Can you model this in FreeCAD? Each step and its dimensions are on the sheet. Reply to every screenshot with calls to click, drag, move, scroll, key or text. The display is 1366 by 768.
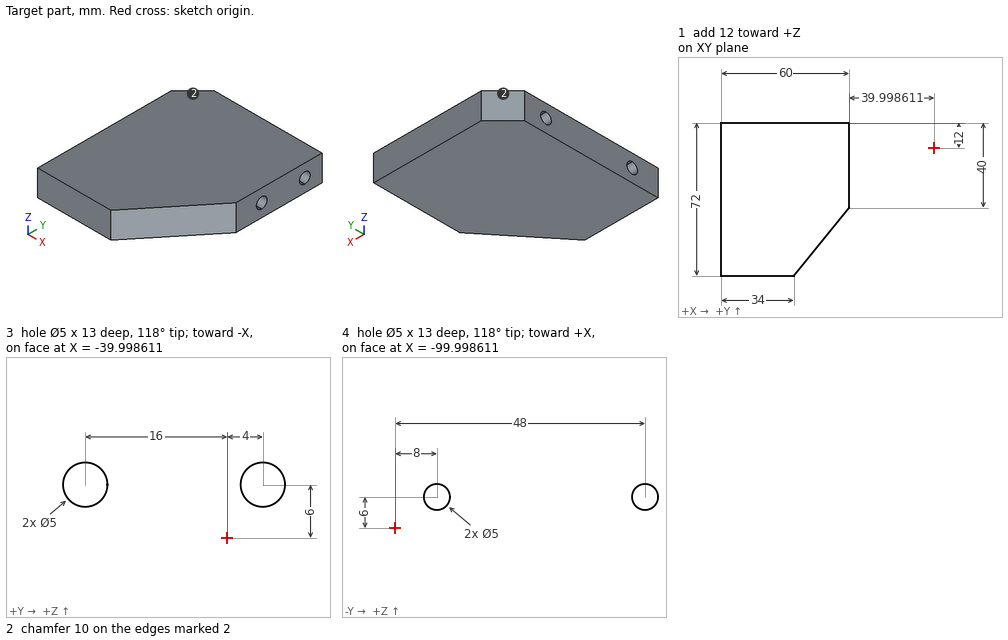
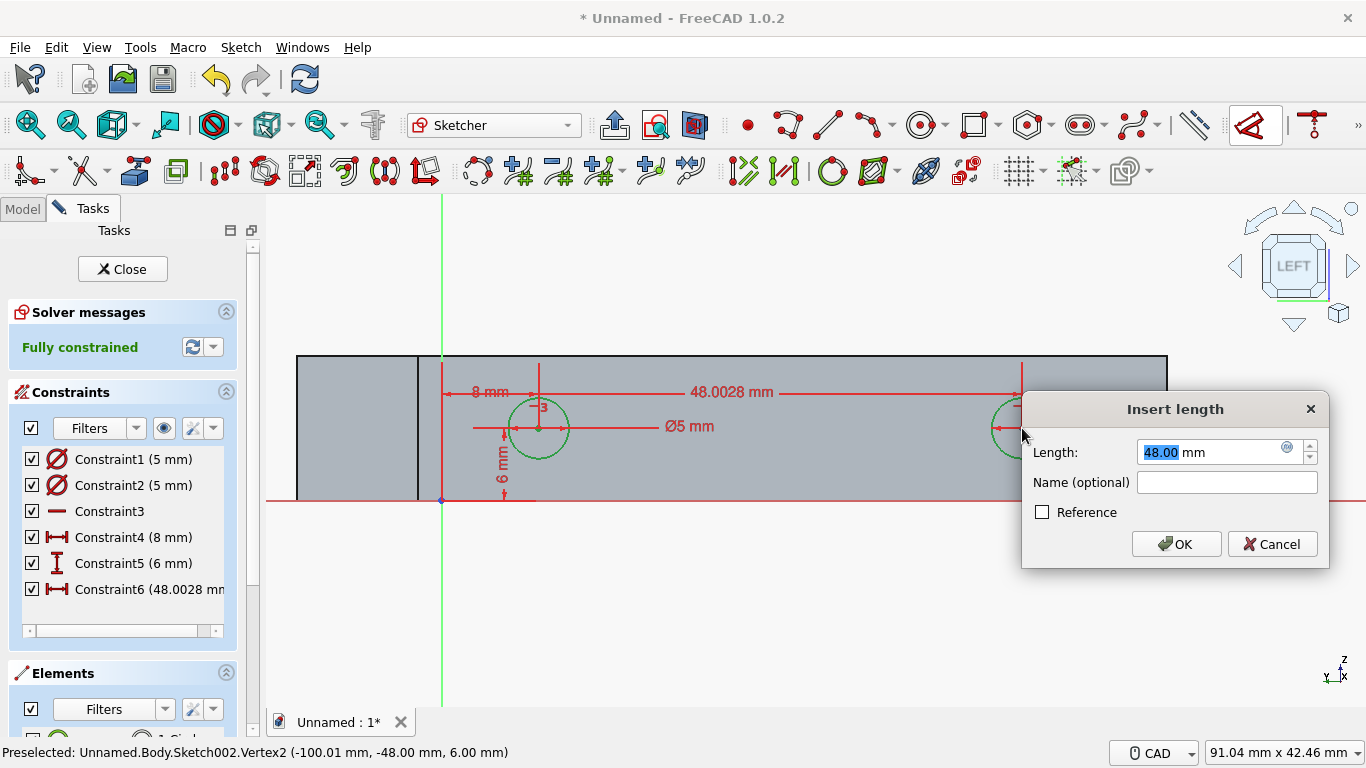
text(48)
key(Return)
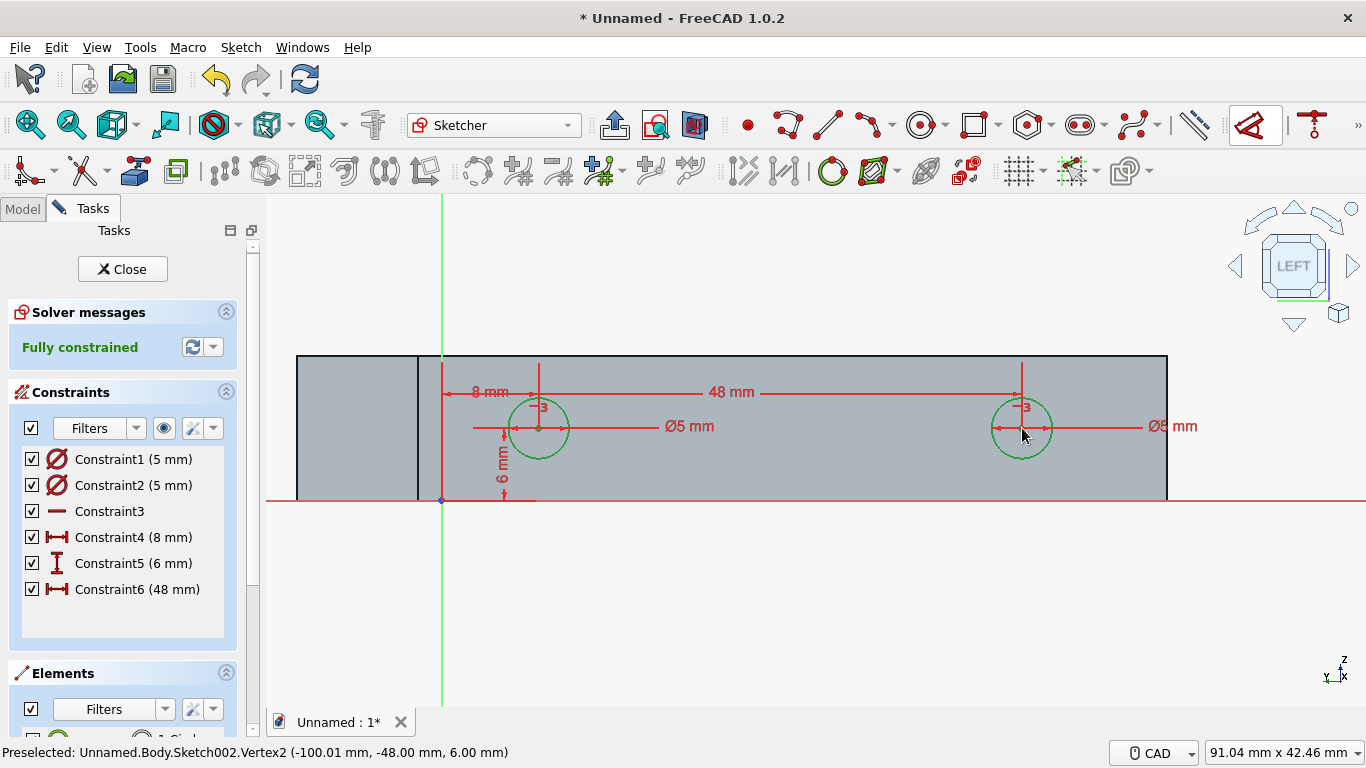
click(123, 269)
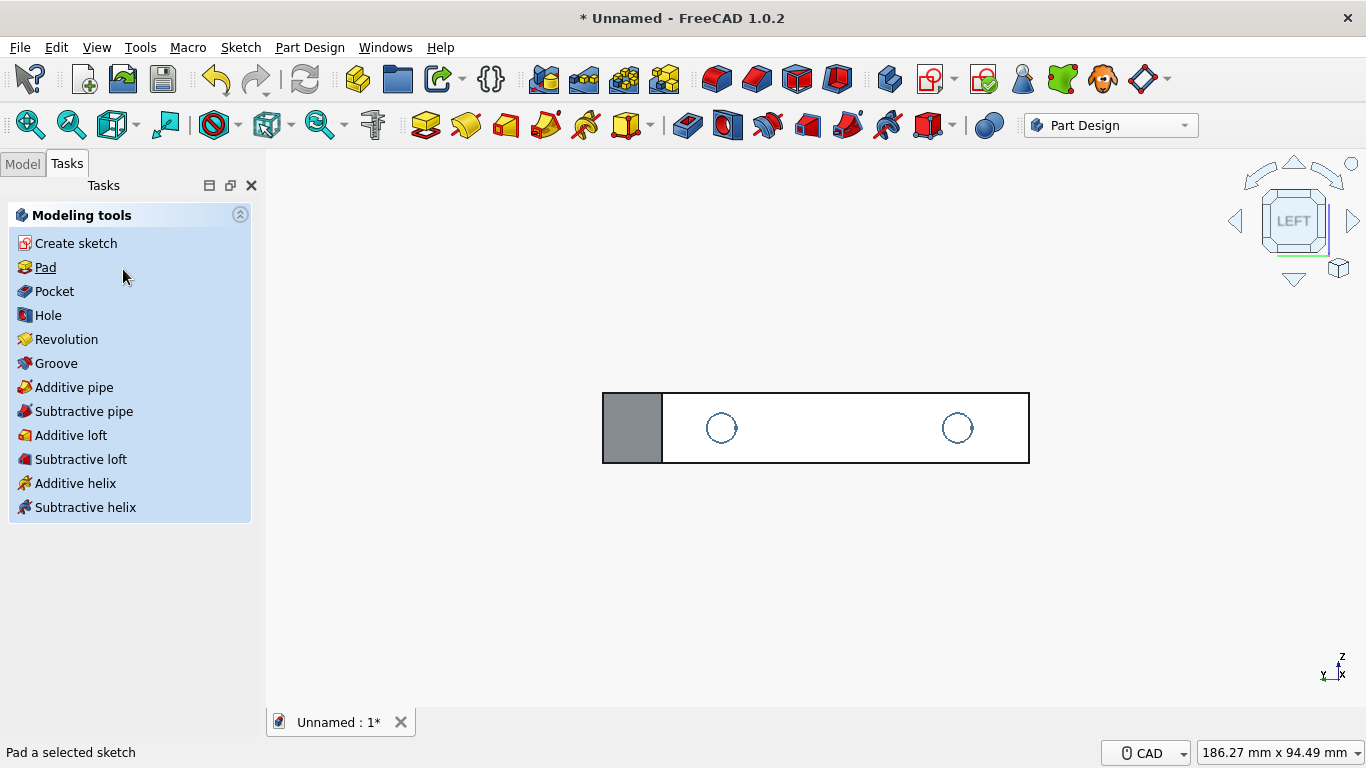
click(728, 126)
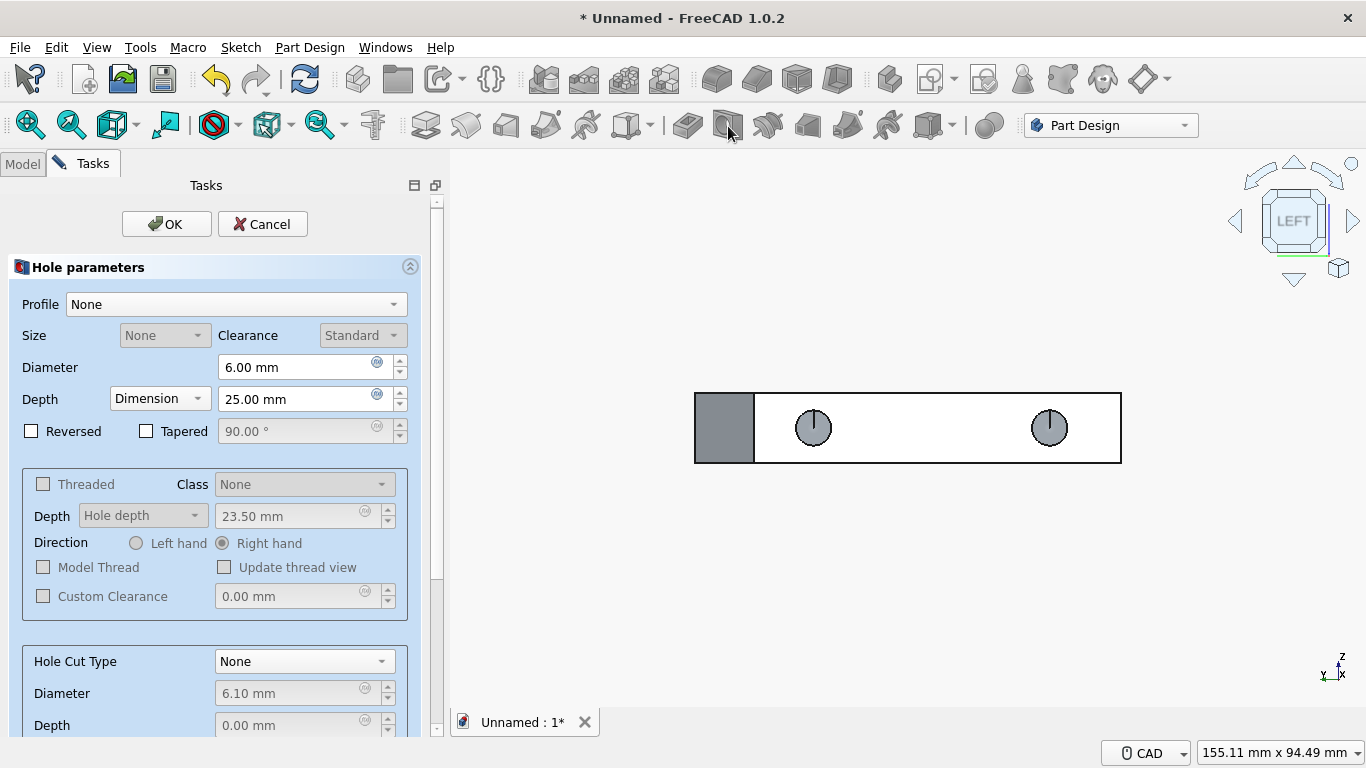
triple_click(305, 367)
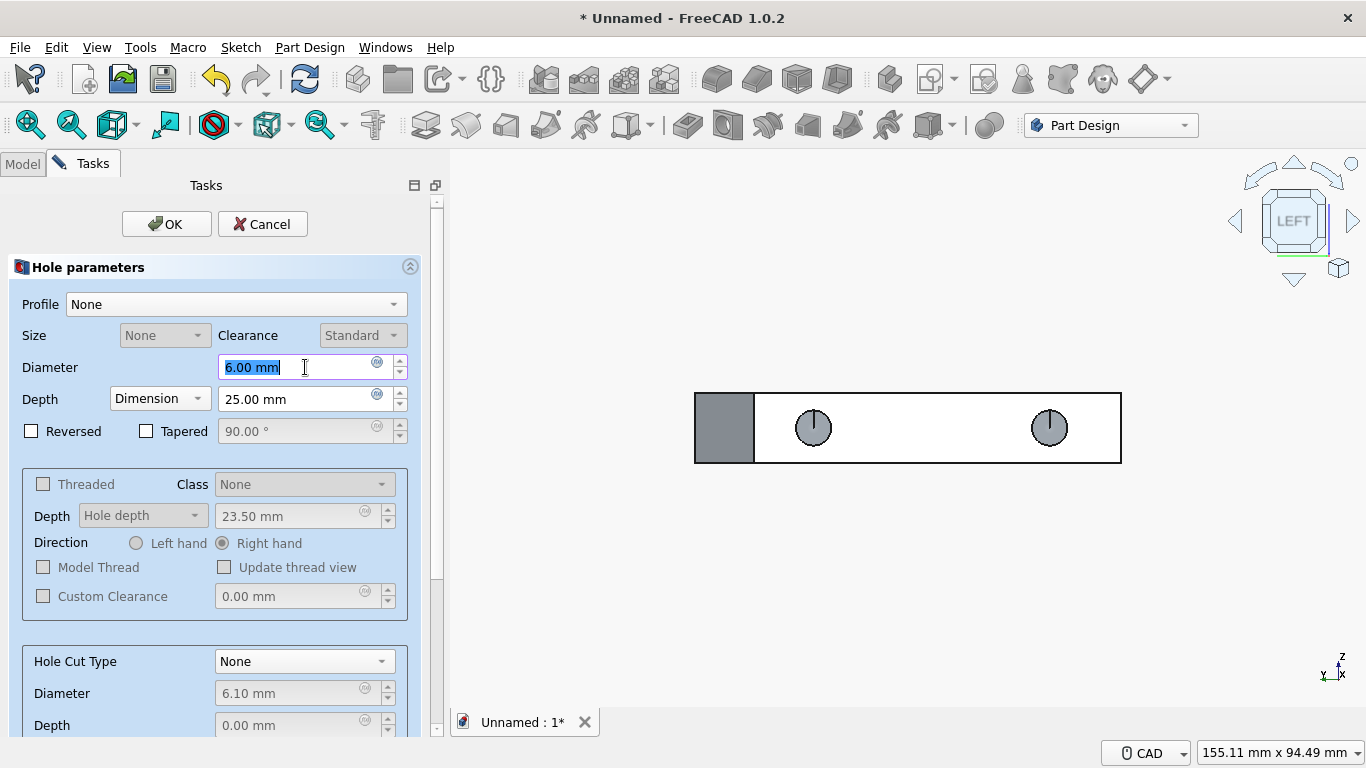
text(5)
key(Tab)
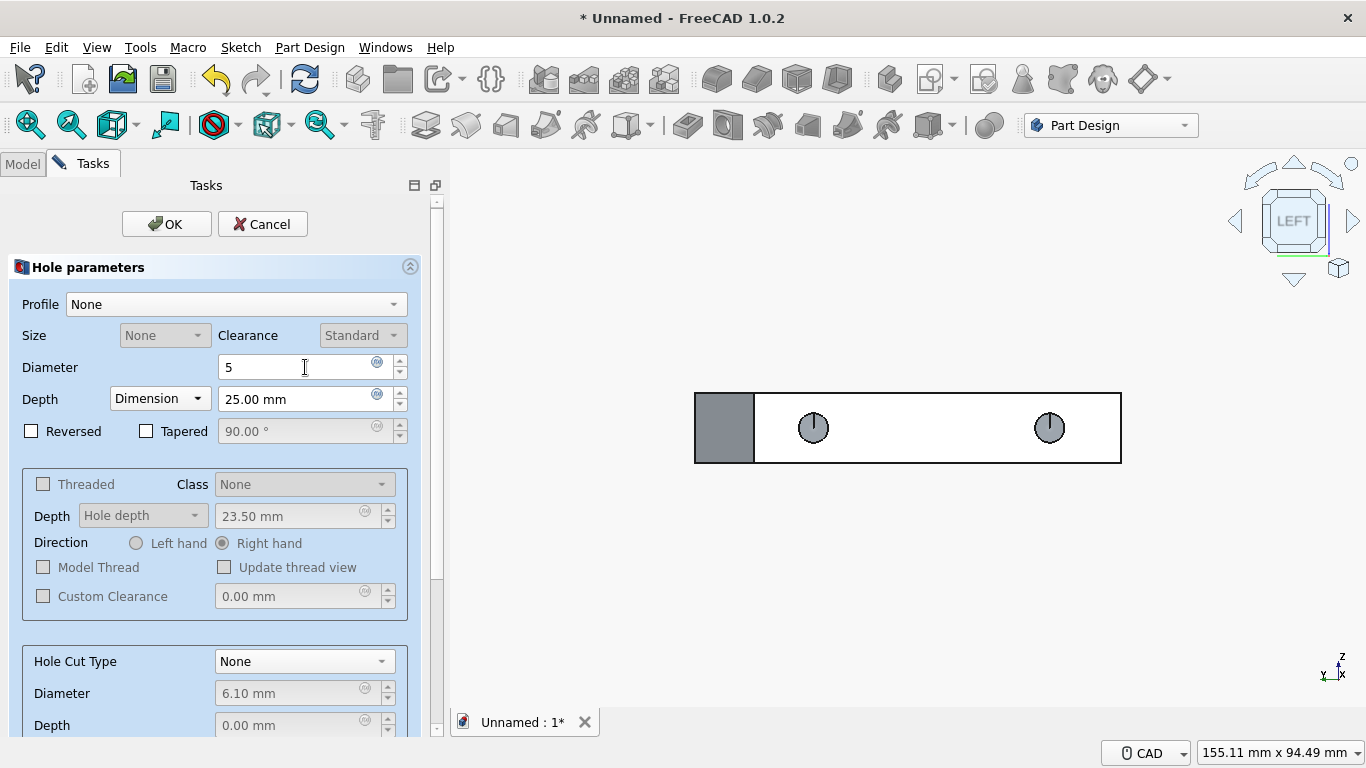
triple_click(305, 399)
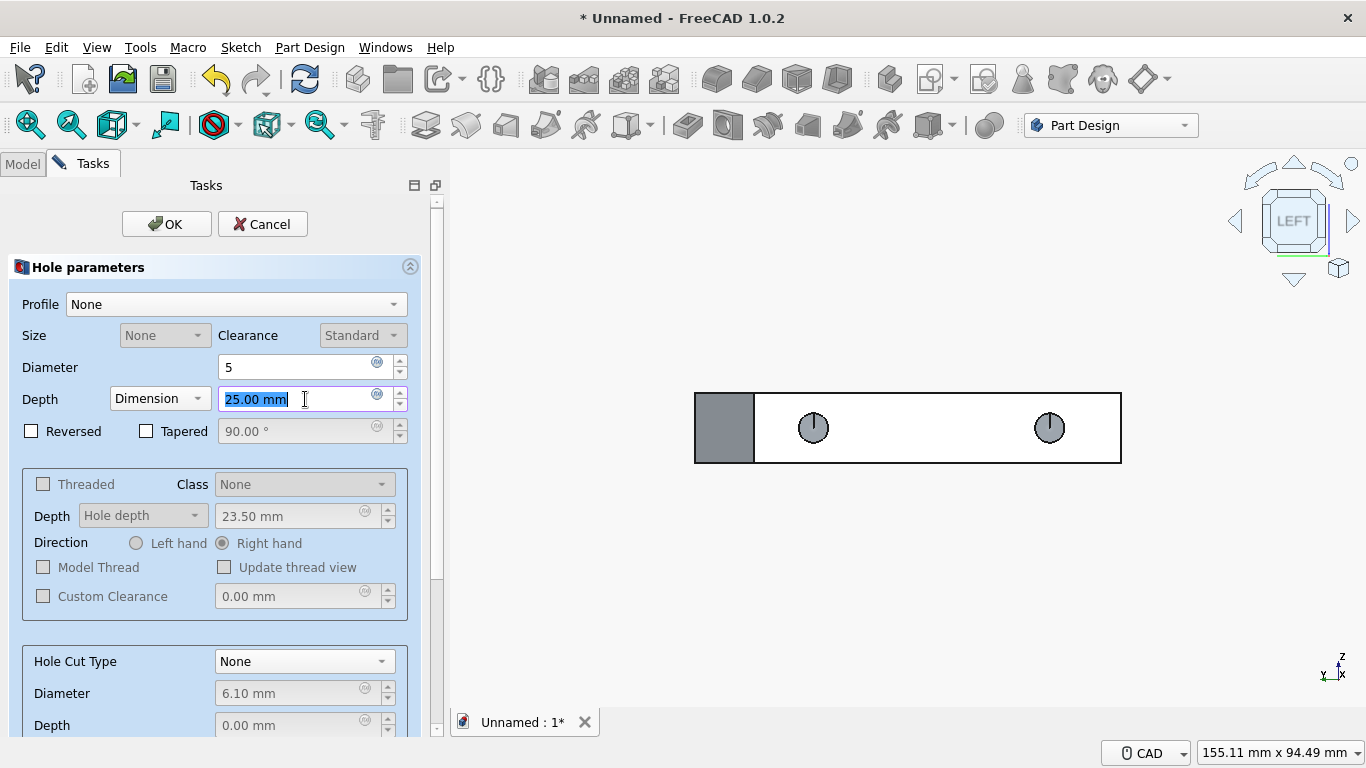
text(13)
key(Tab)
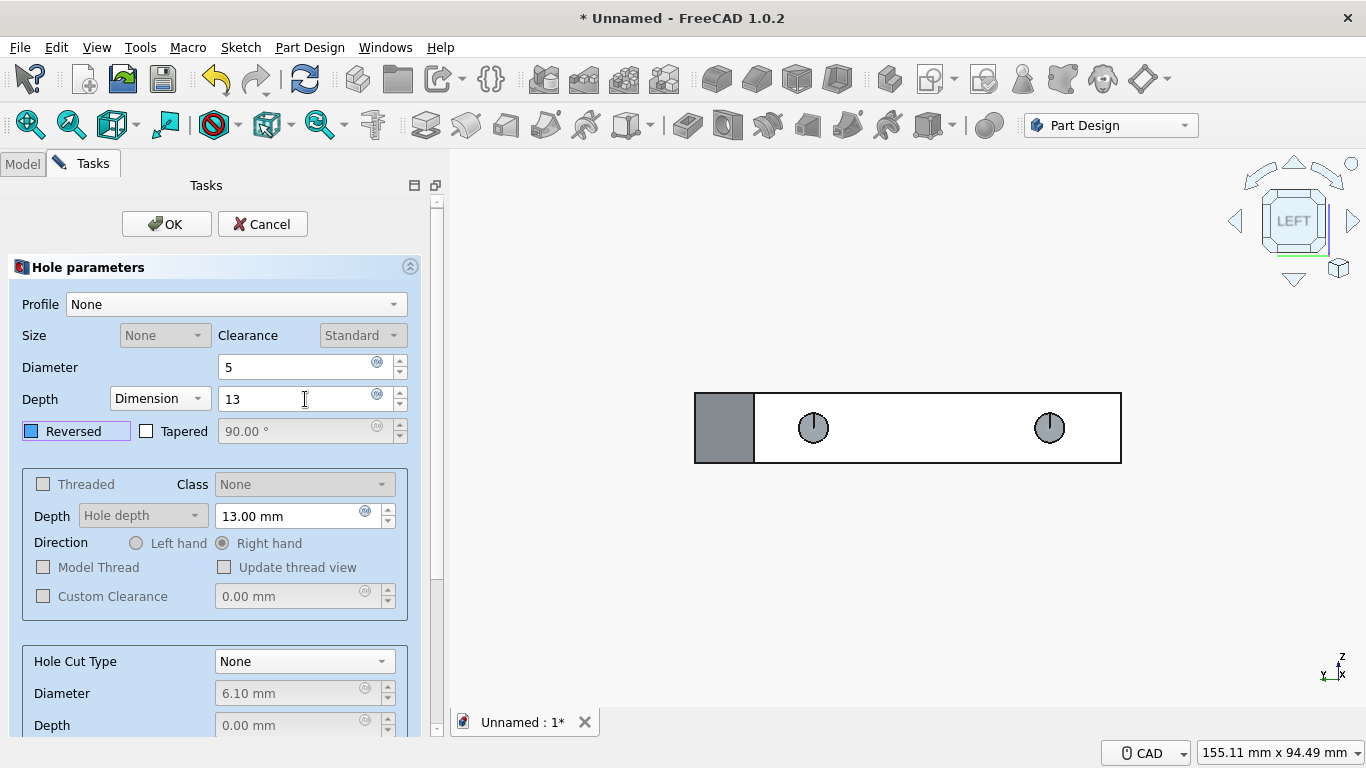
click(167, 224)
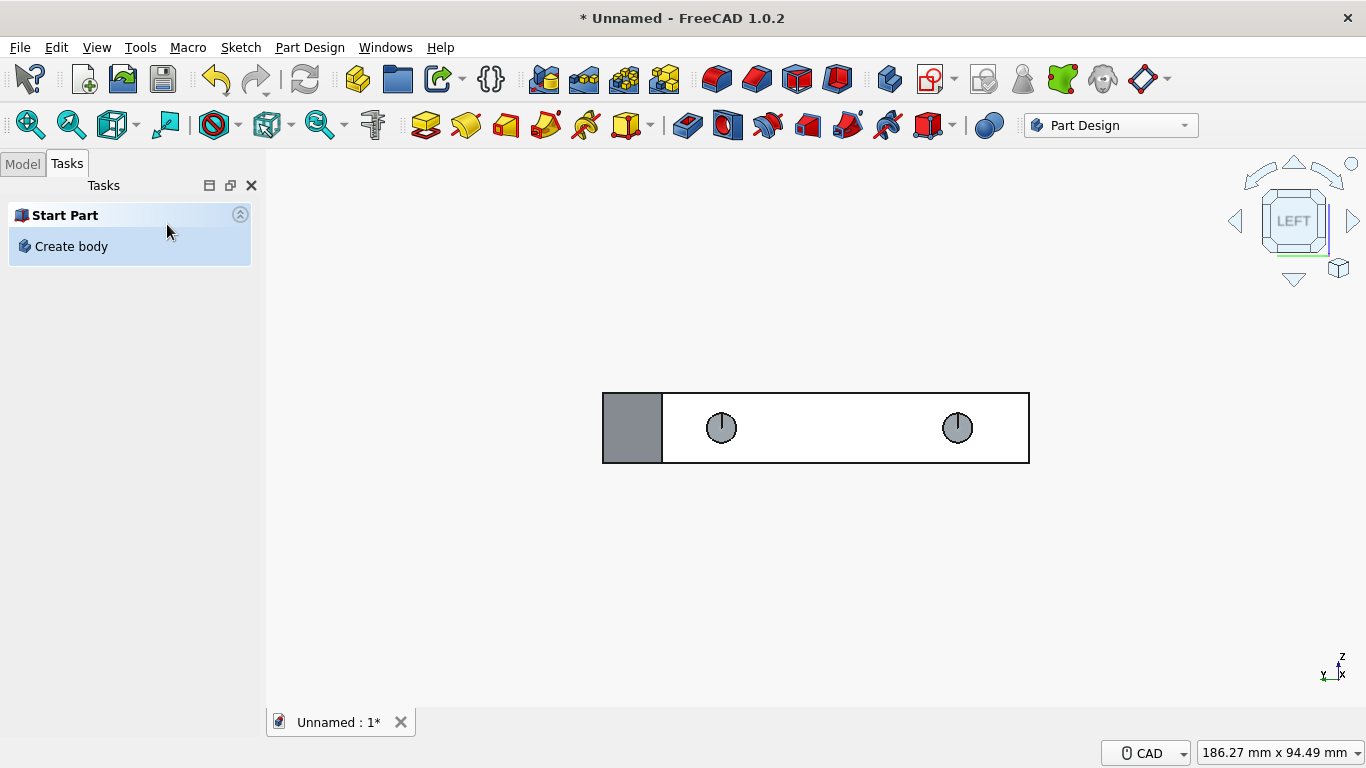
key(0)